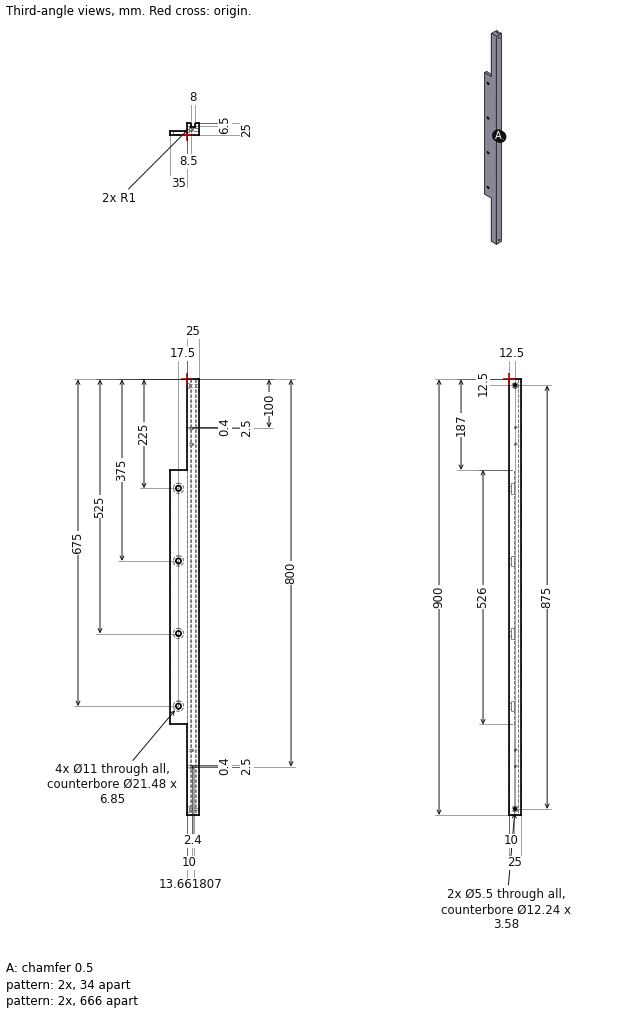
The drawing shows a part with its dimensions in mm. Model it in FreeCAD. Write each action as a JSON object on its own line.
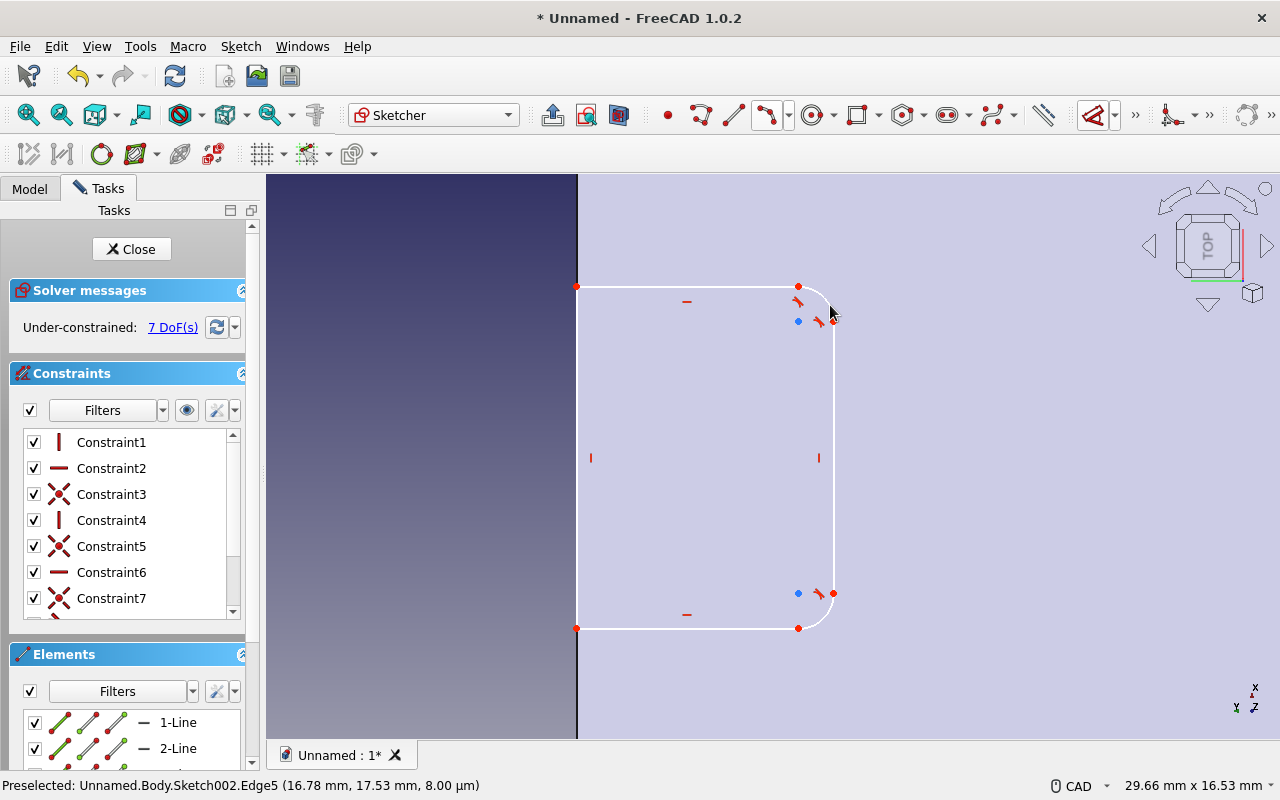
{"action": "left_click", "coordinate": [644, 629]}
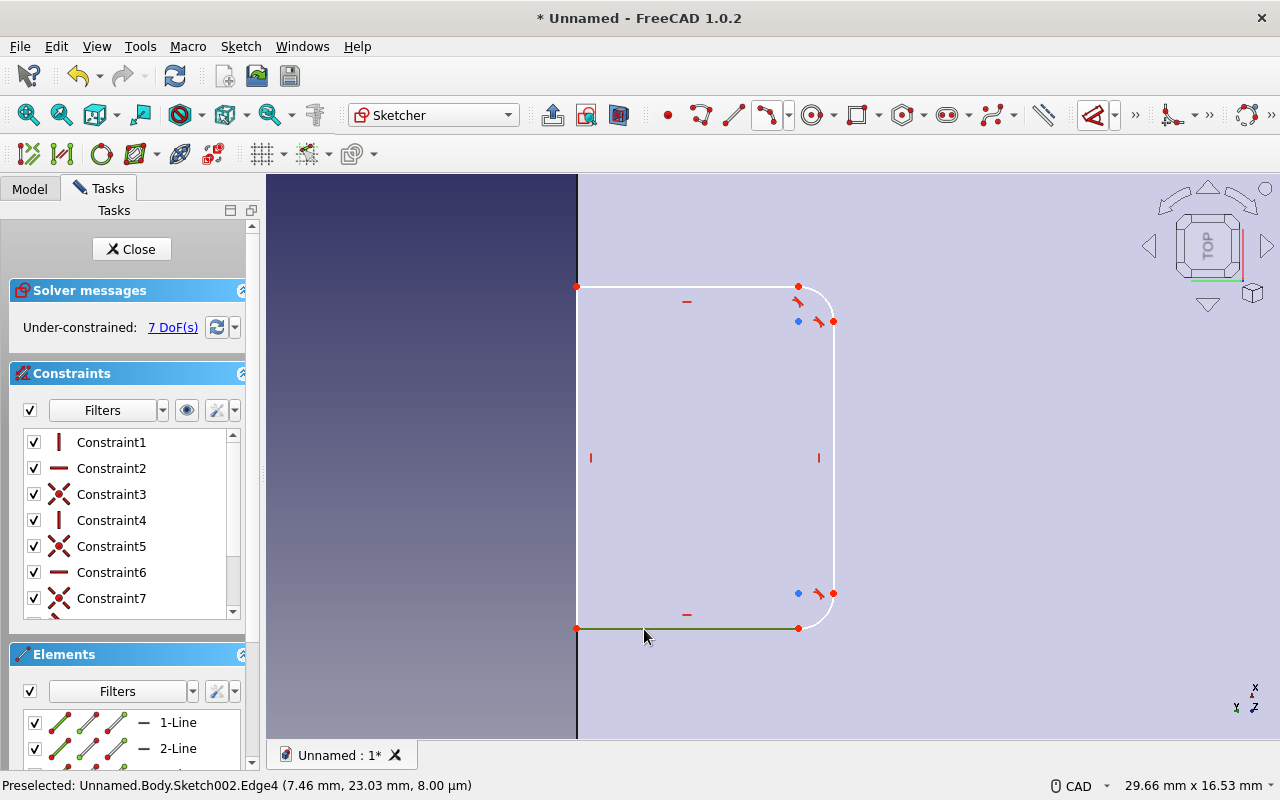
{"action": "left_click", "coordinate": [815, 625]}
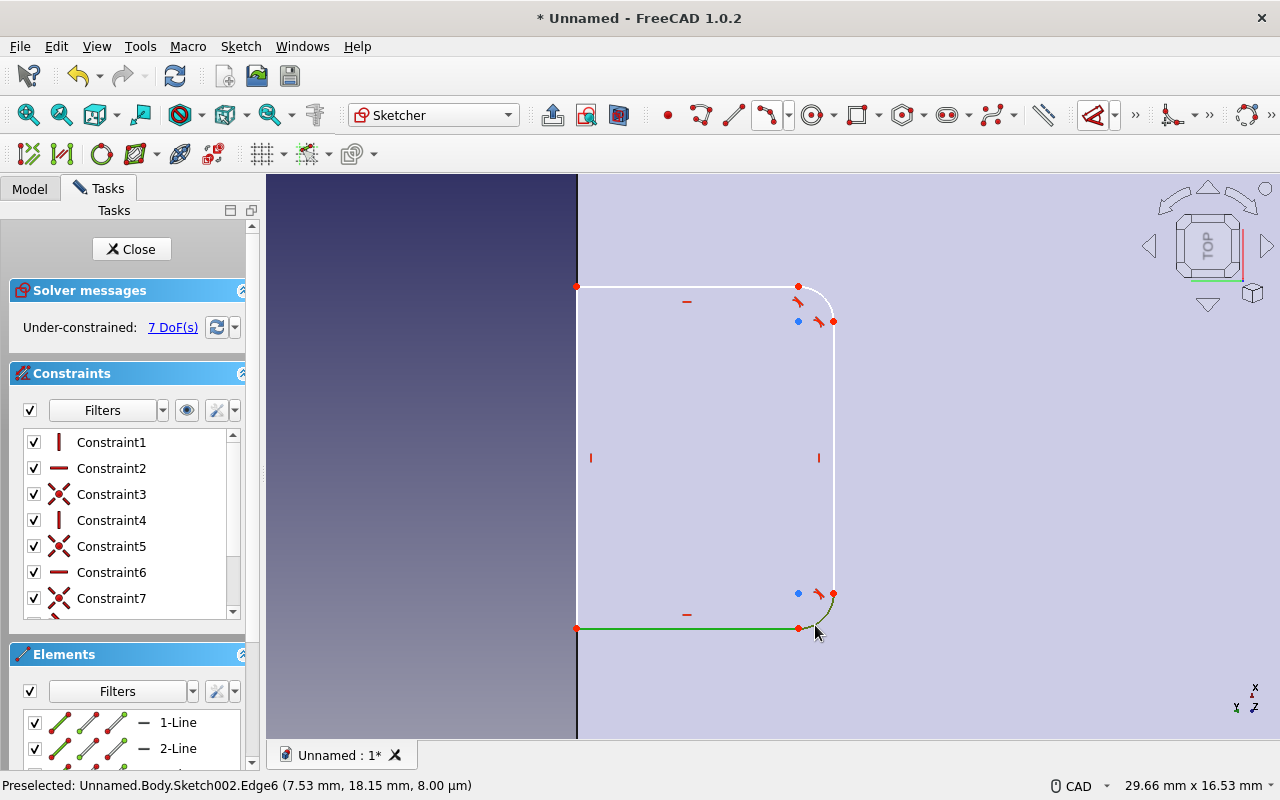
{"action": "key", "text": "t"}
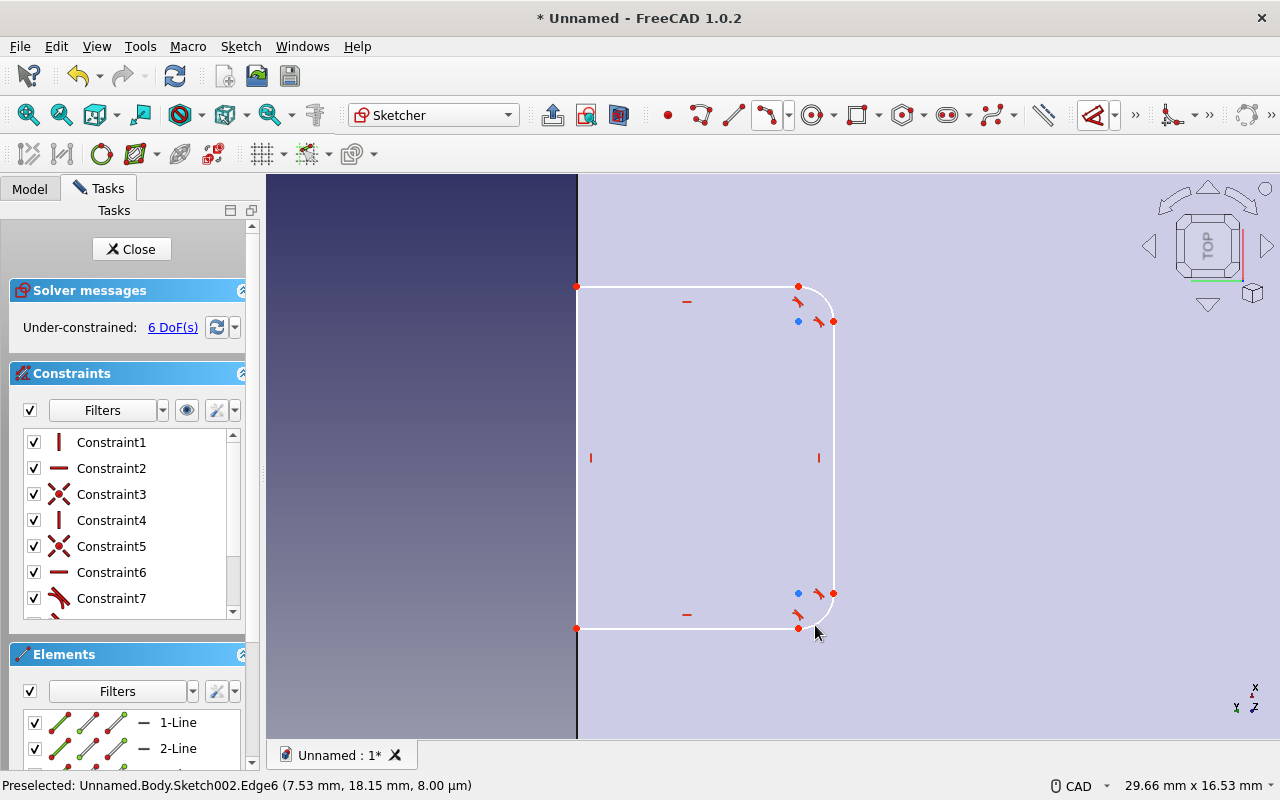
{"action": "left_click", "coordinate": [830, 306]}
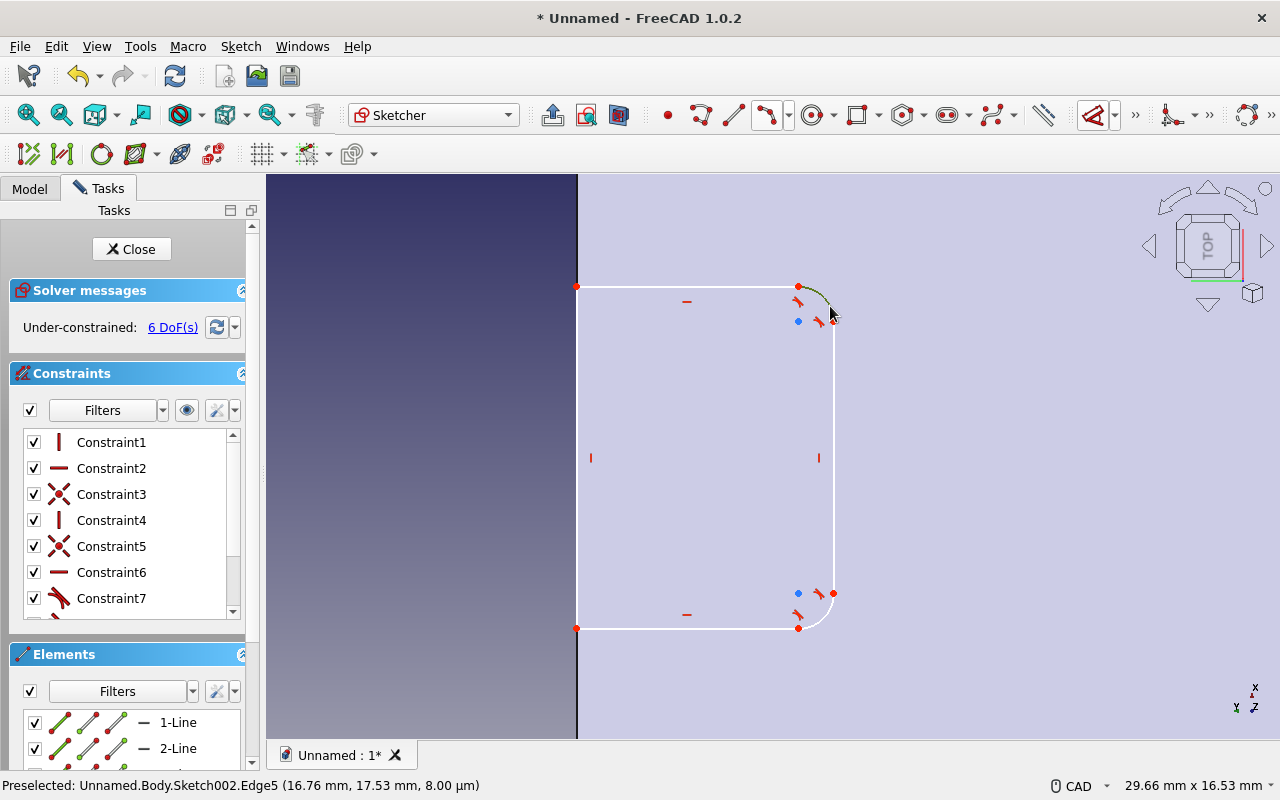
{"action": "left_click", "coordinate": [814, 625]}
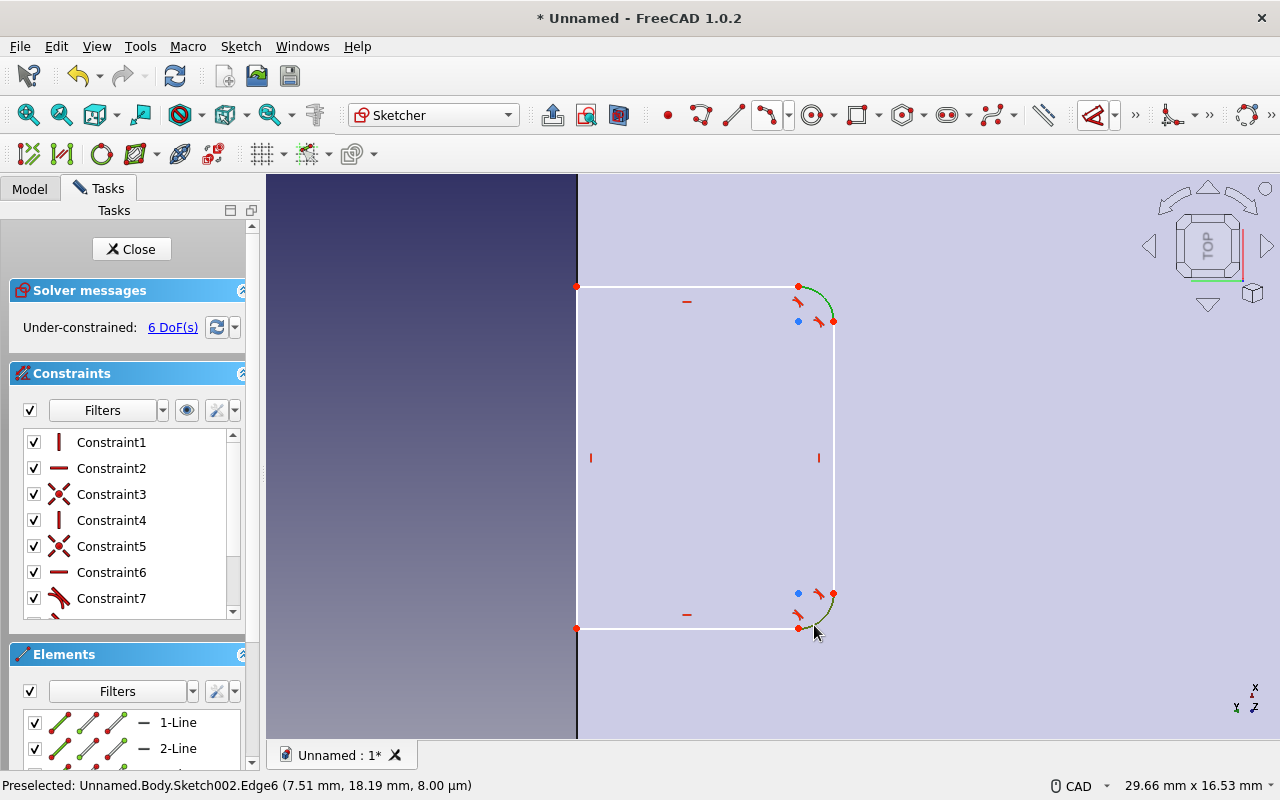
{"action": "key", "text": "e"}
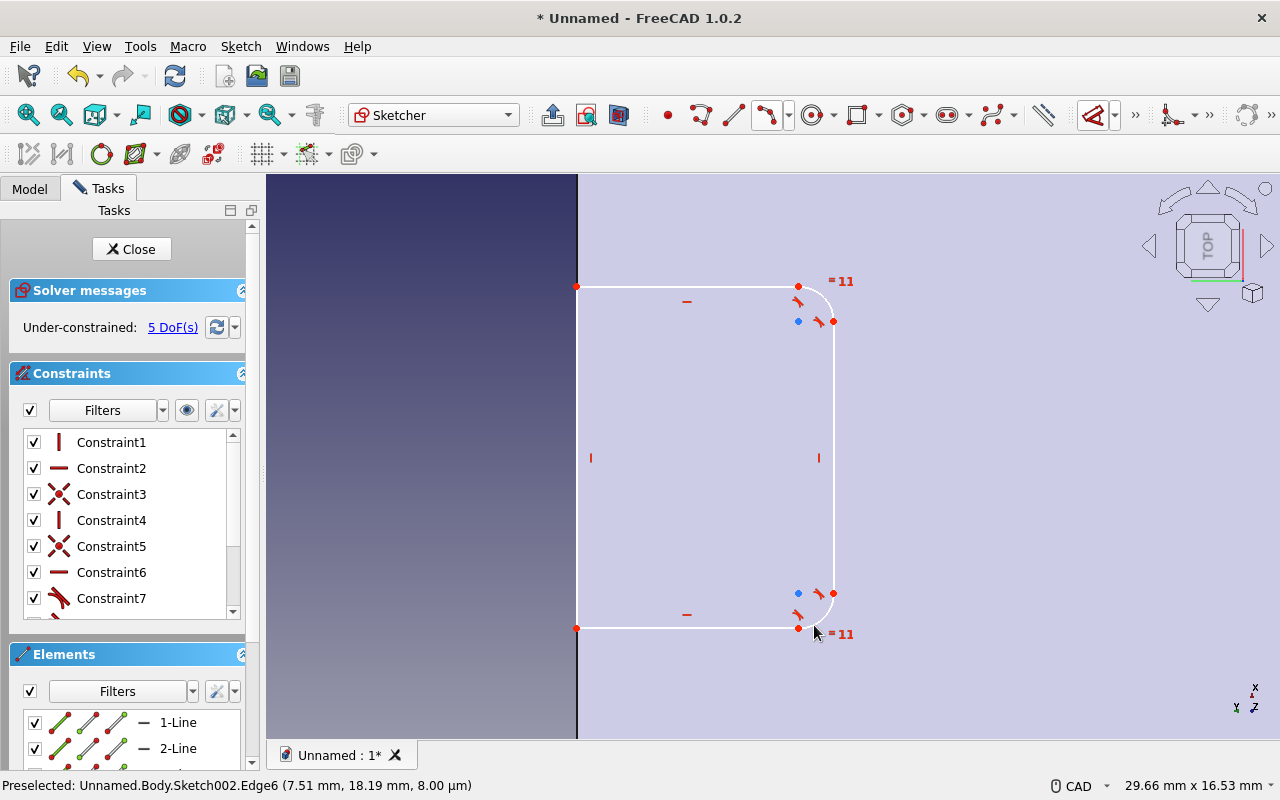
{"action": "left_click", "coordinate": [830, 306]}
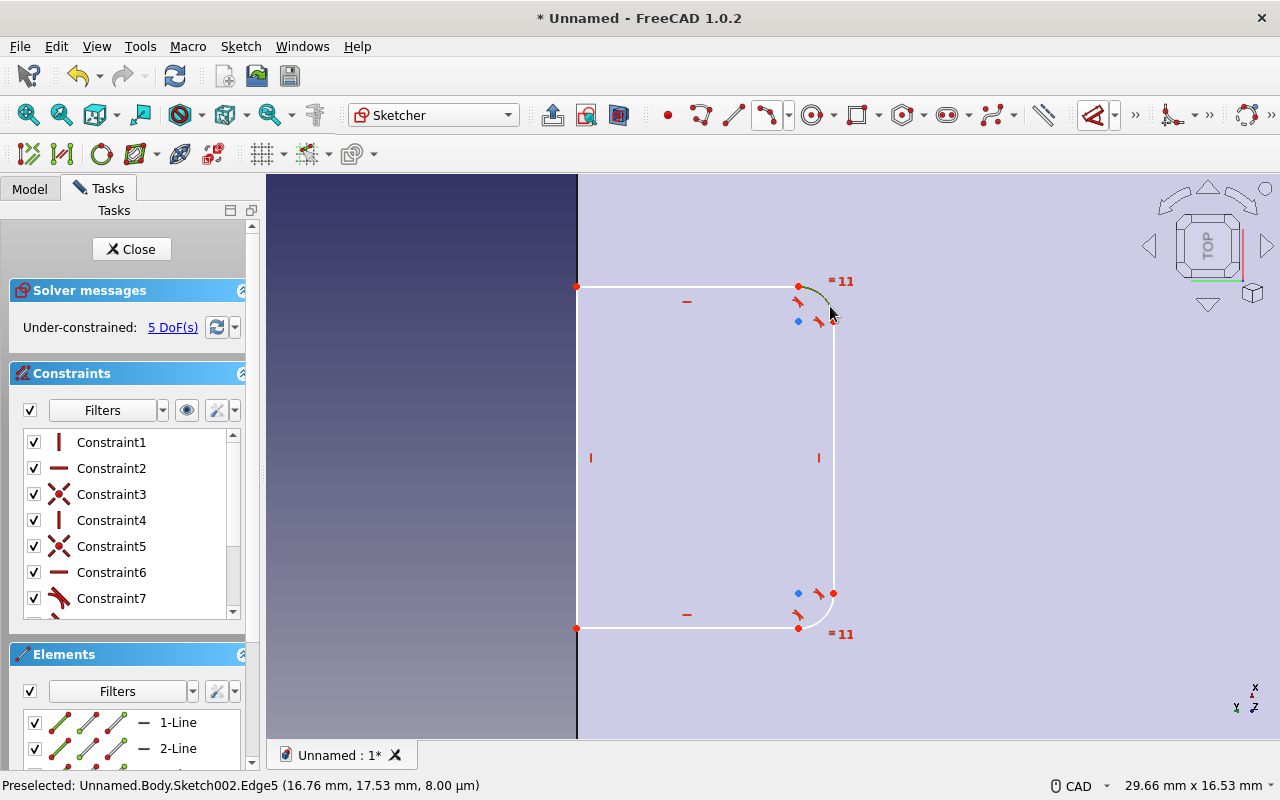
{"action": "left_click", "coordinate": [1114, 116]}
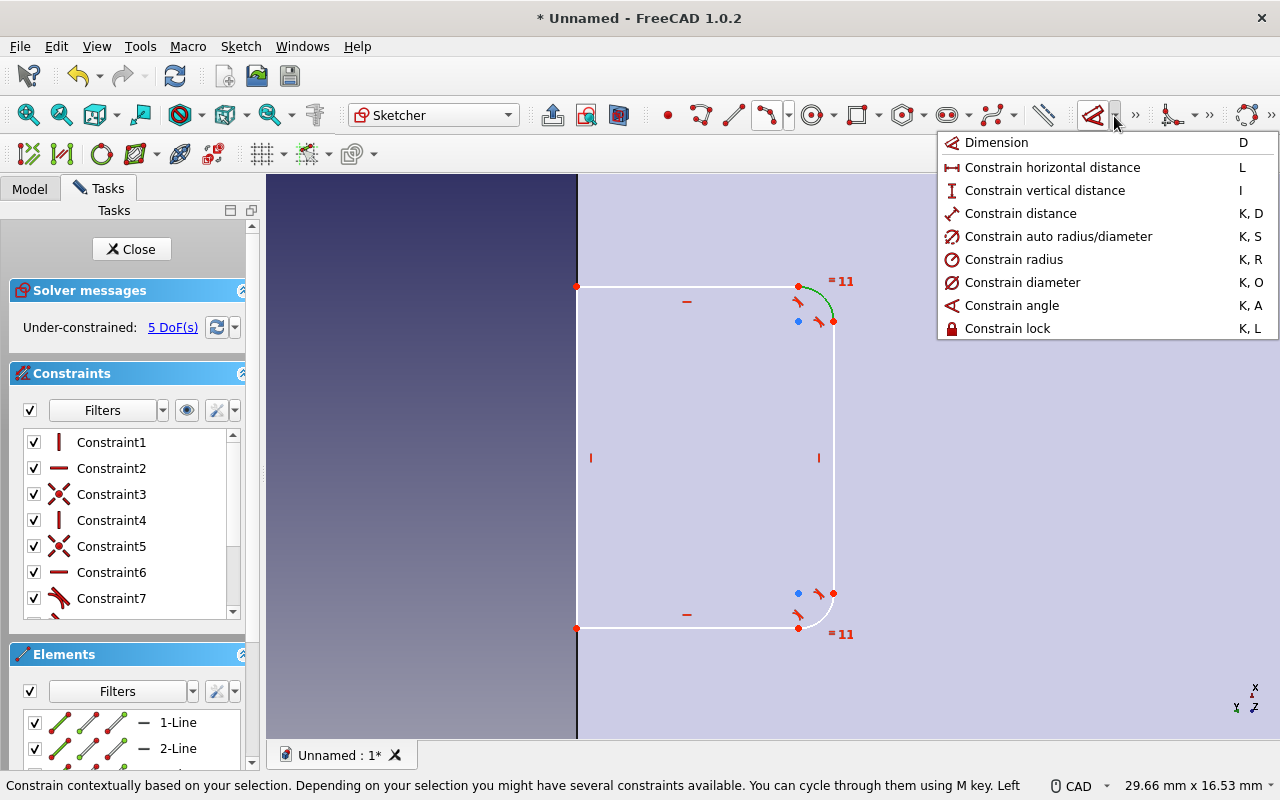
{"action": "left_click", "coordinate": [1108, 260]}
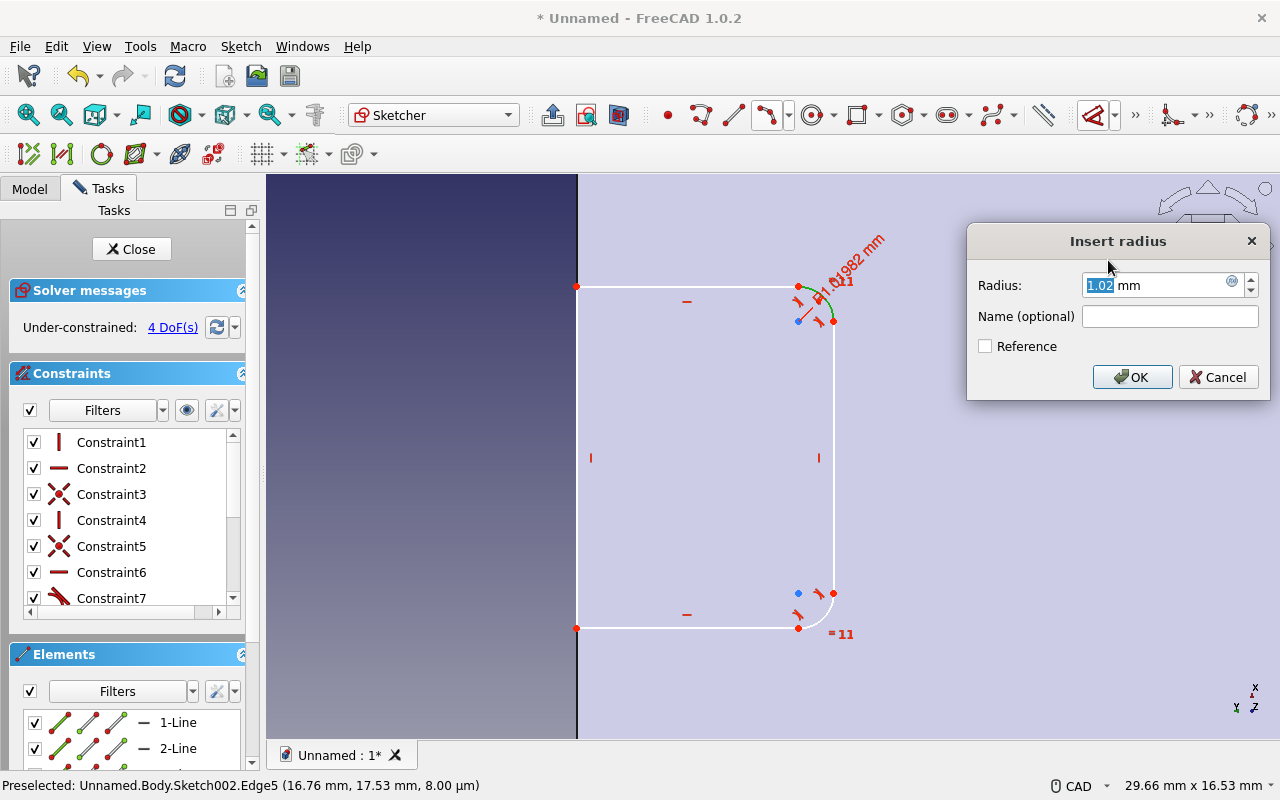
{"action": "type", "text": "1"}
{"action": "key", "text": "Return"}